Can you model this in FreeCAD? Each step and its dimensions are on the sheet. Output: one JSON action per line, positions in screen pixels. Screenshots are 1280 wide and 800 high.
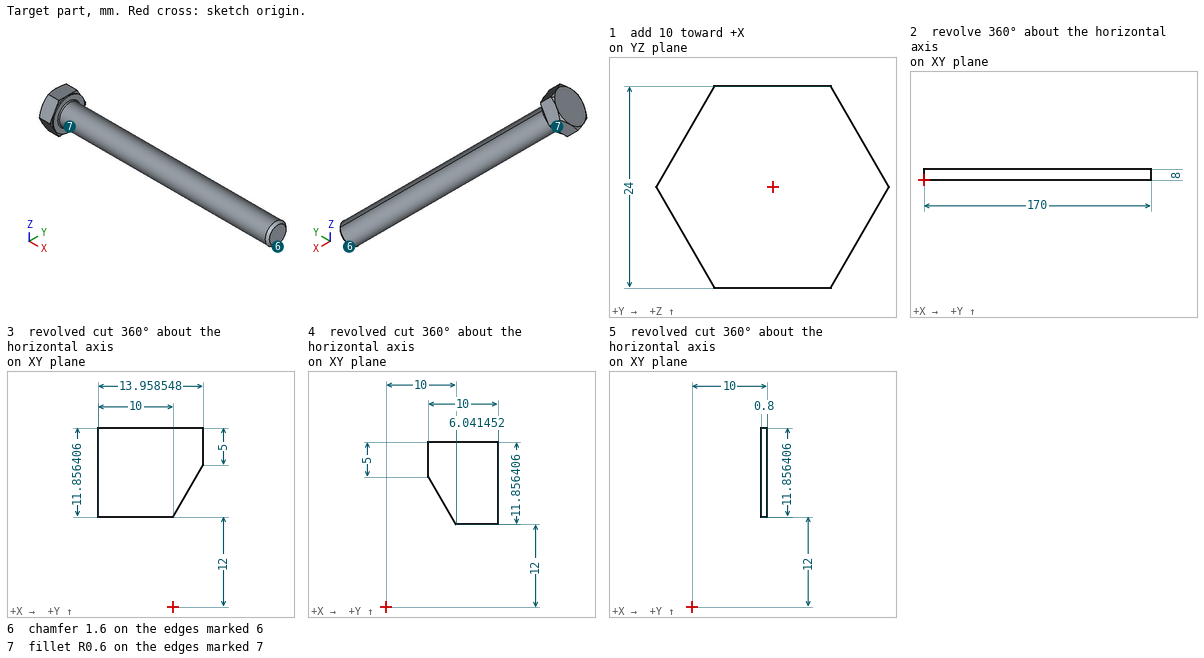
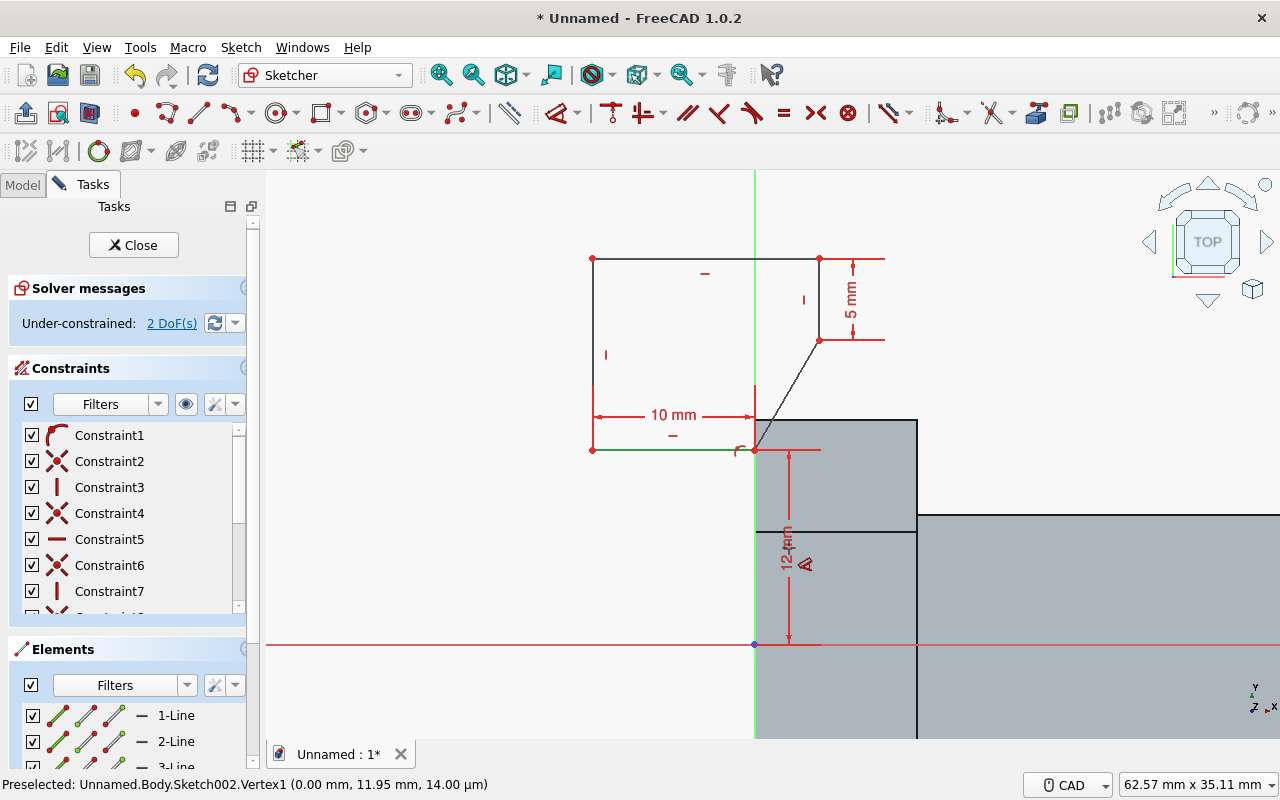
{"action": "left_click", "coordinate": [751, 259]}
{"action": "left_click", "coordinate": [706, 225]}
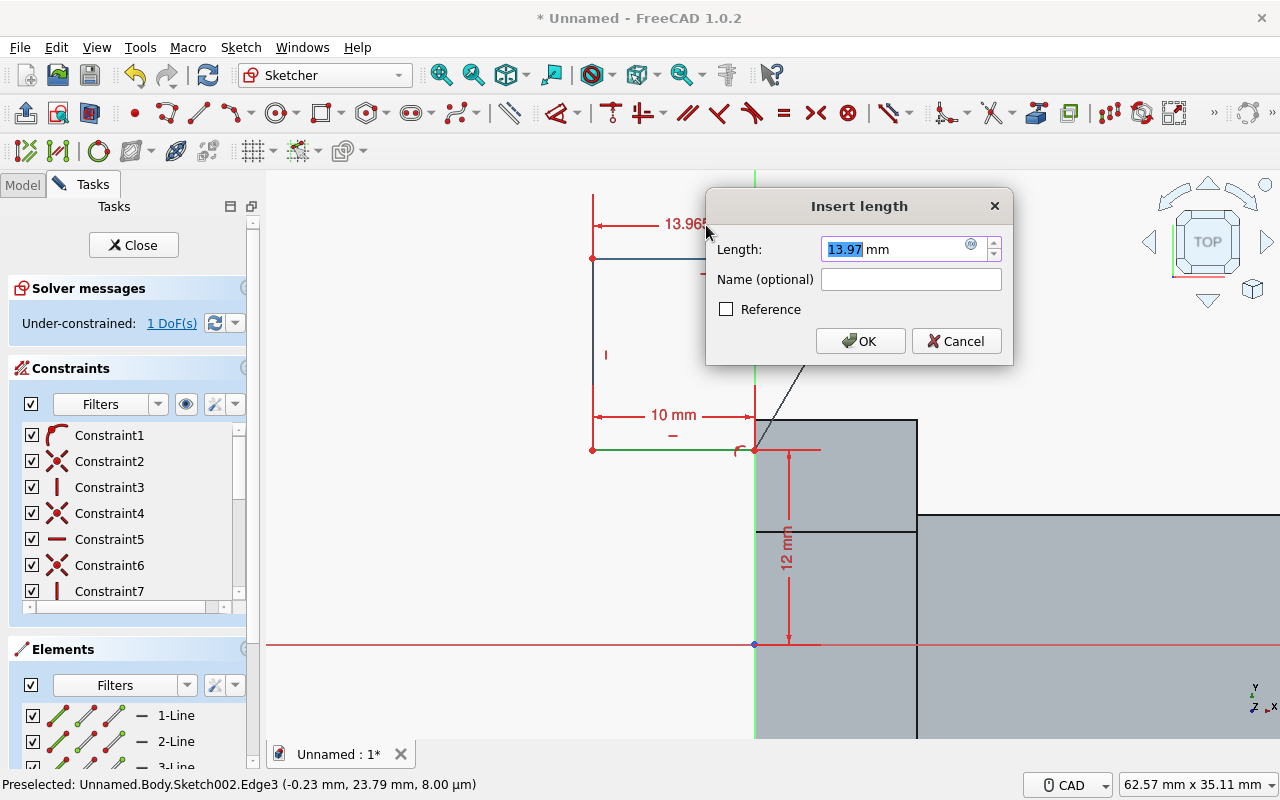
{"action": "type", "text": "13.958548"}
{"action": "key", "text": "Return"}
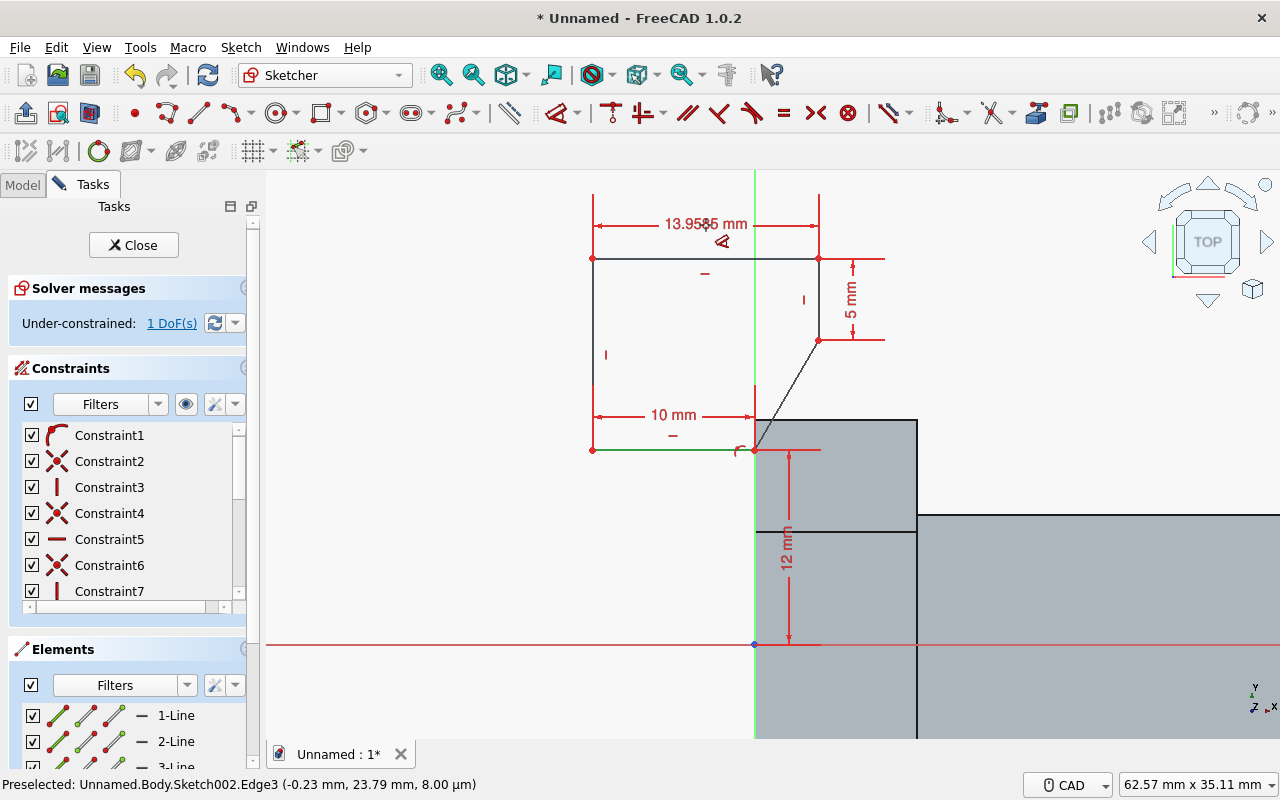
{"action": "left_click", "coordinate": [593, 316]}
{"action": "left_click", "coordinate": [559, 355]}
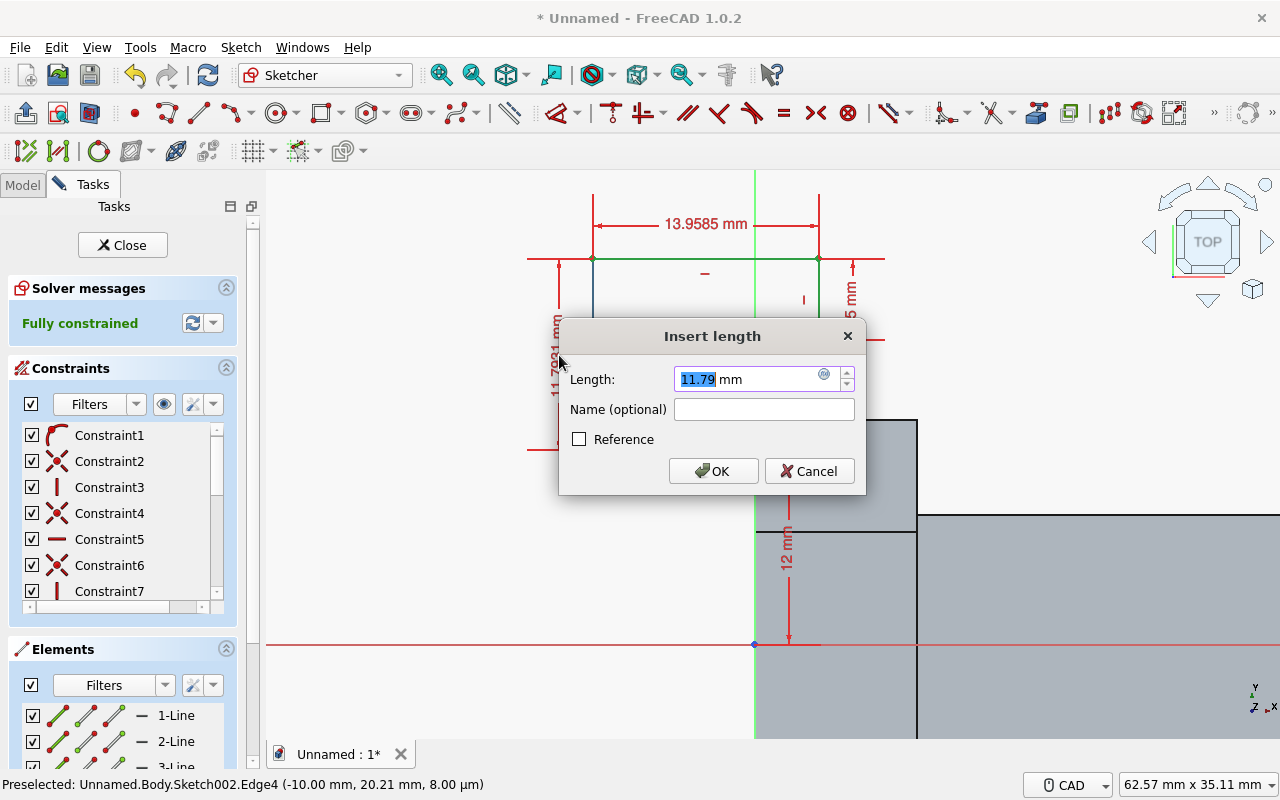
{"action": "type", "text": "11.856406"}
{"action": "key", "text": "Return"}
{"action": "key", "text": "Escape"}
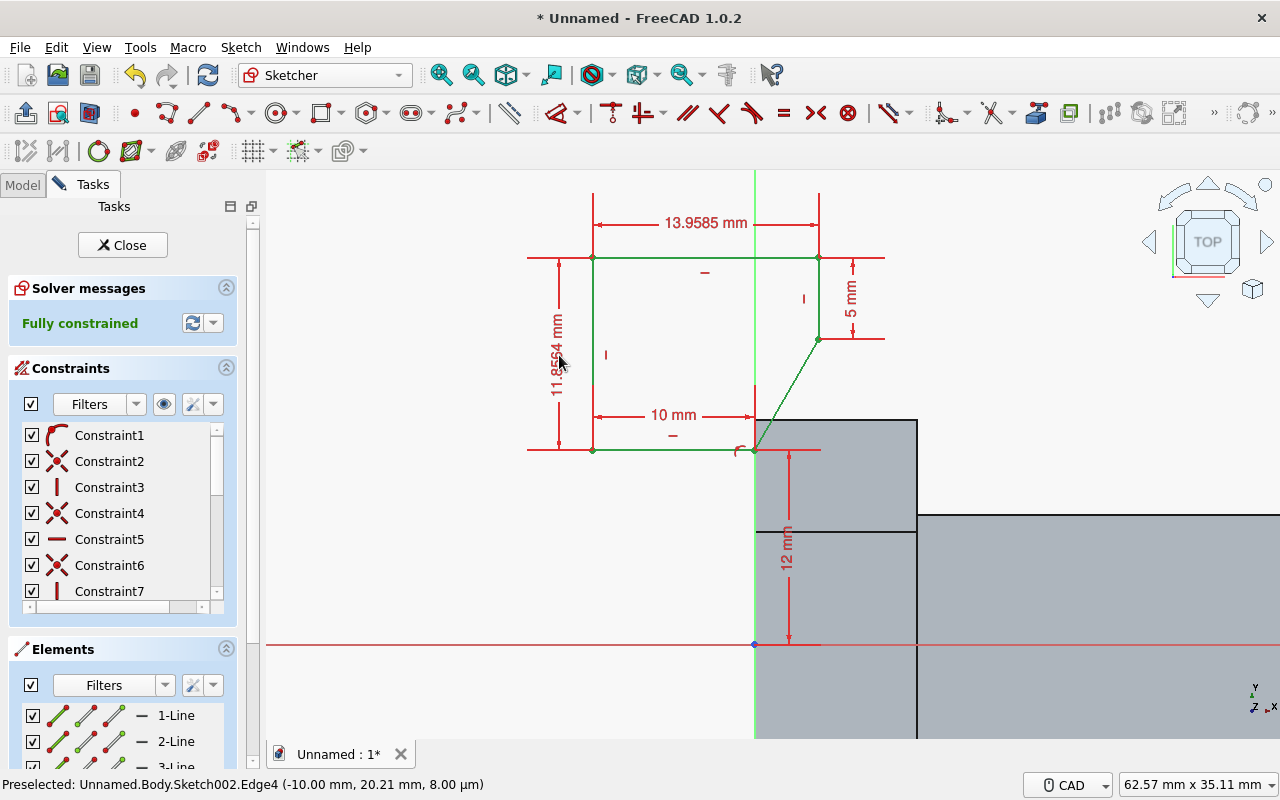
{"action": "left_click", "coordinate": [123, 245]}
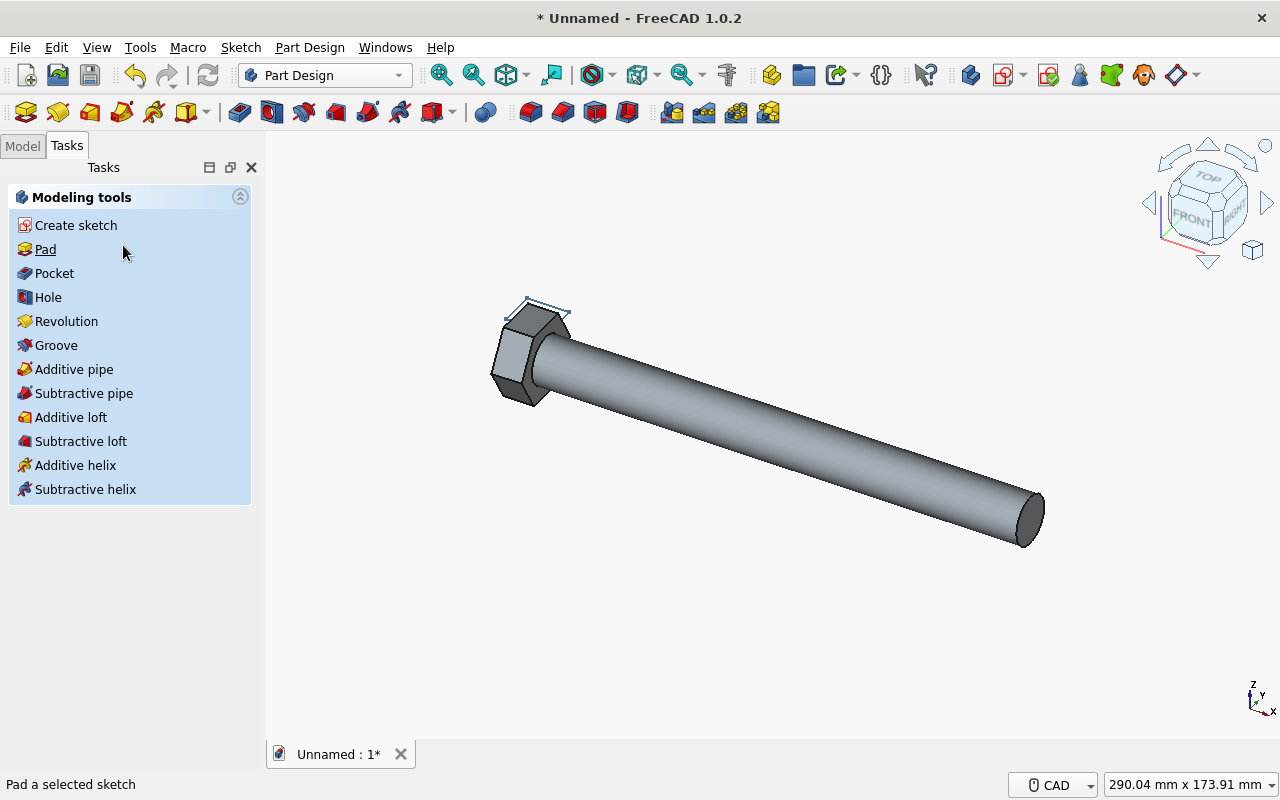
{"action": "left_click", "coordinate": [304, 112]}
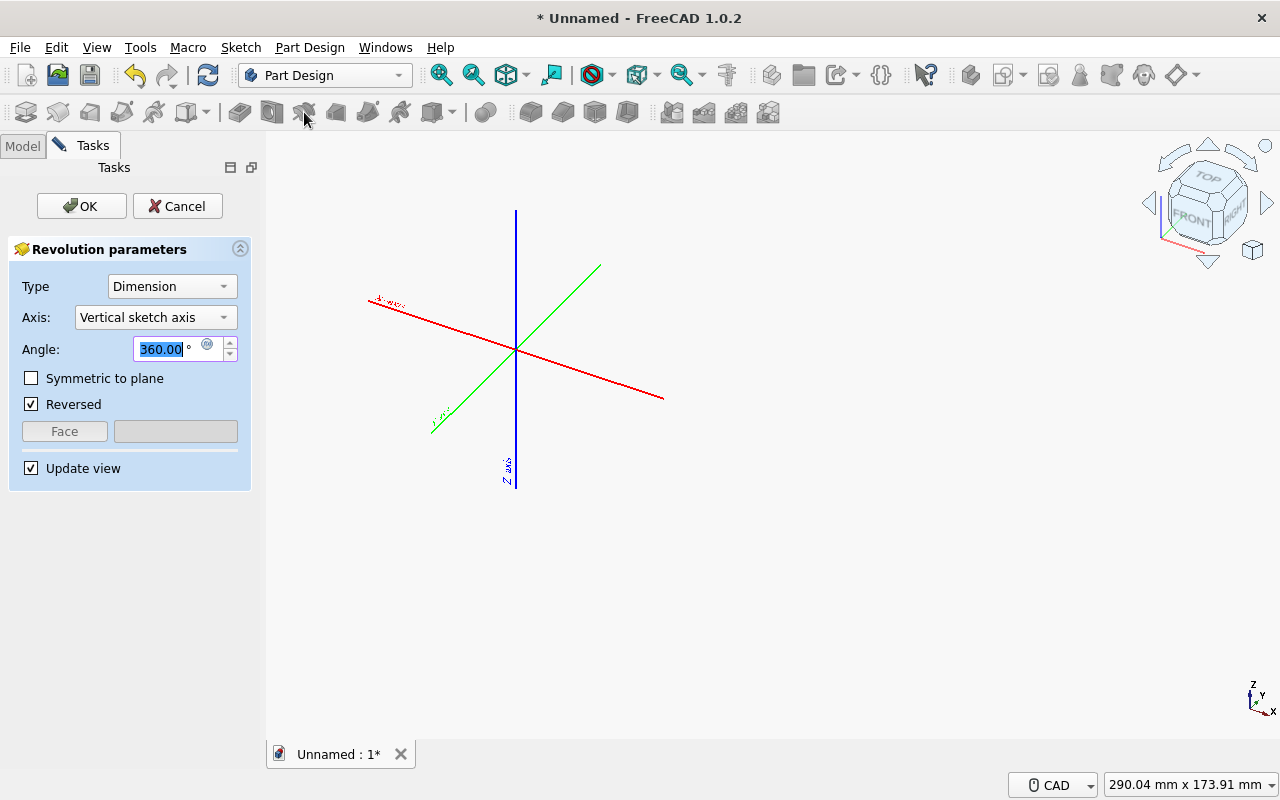
{"action": "left_click", "coordinate": [156, 318]}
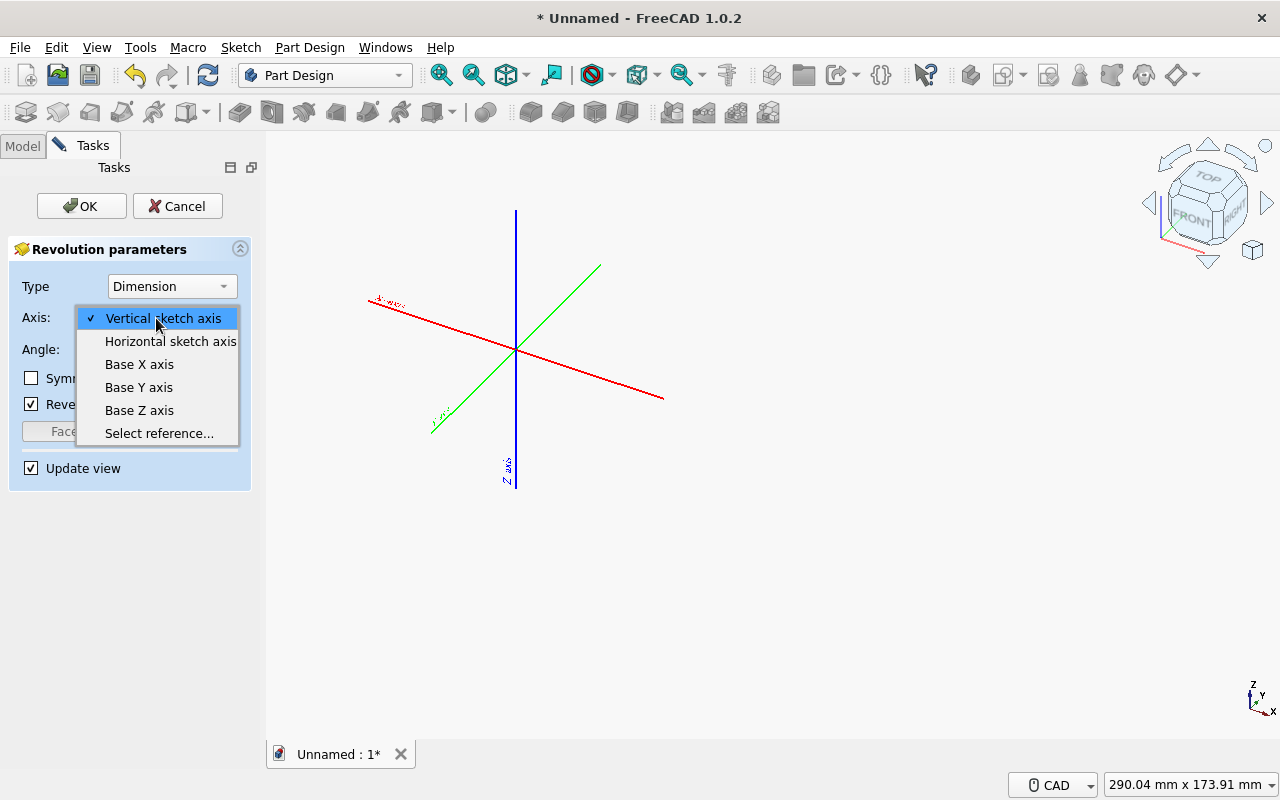
{"action": "left_click", "coordinate": [156, 342]}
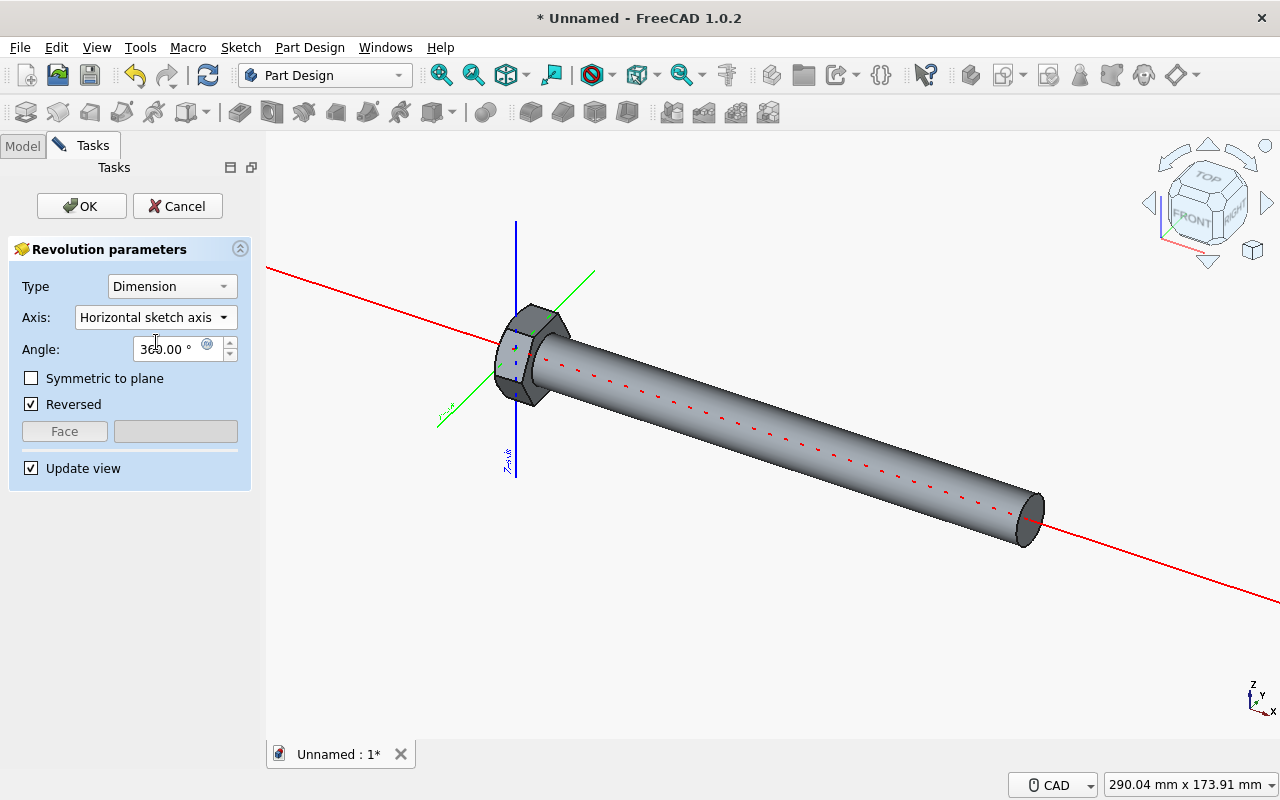
{"action": "left_click", "coordinate": [82, 206]}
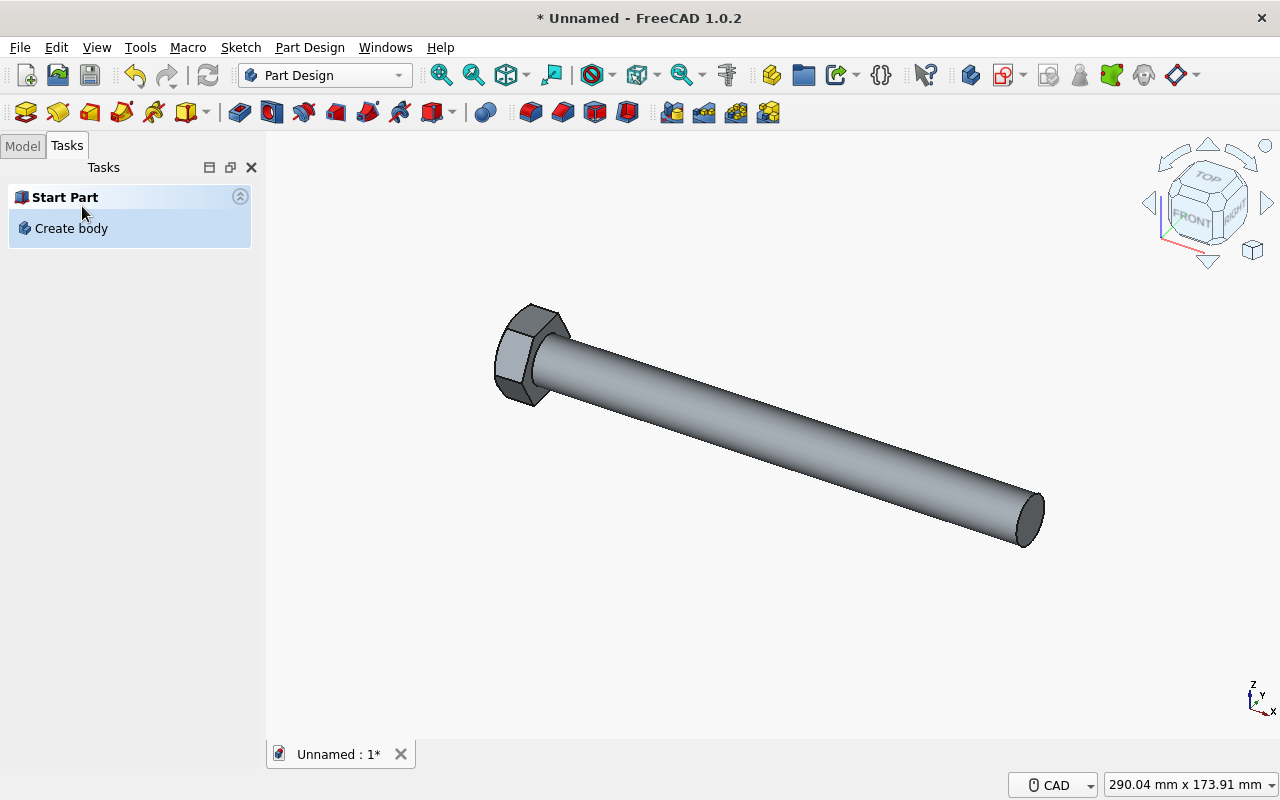
{"action": "left_click", "coordinate": [1004, 76]}